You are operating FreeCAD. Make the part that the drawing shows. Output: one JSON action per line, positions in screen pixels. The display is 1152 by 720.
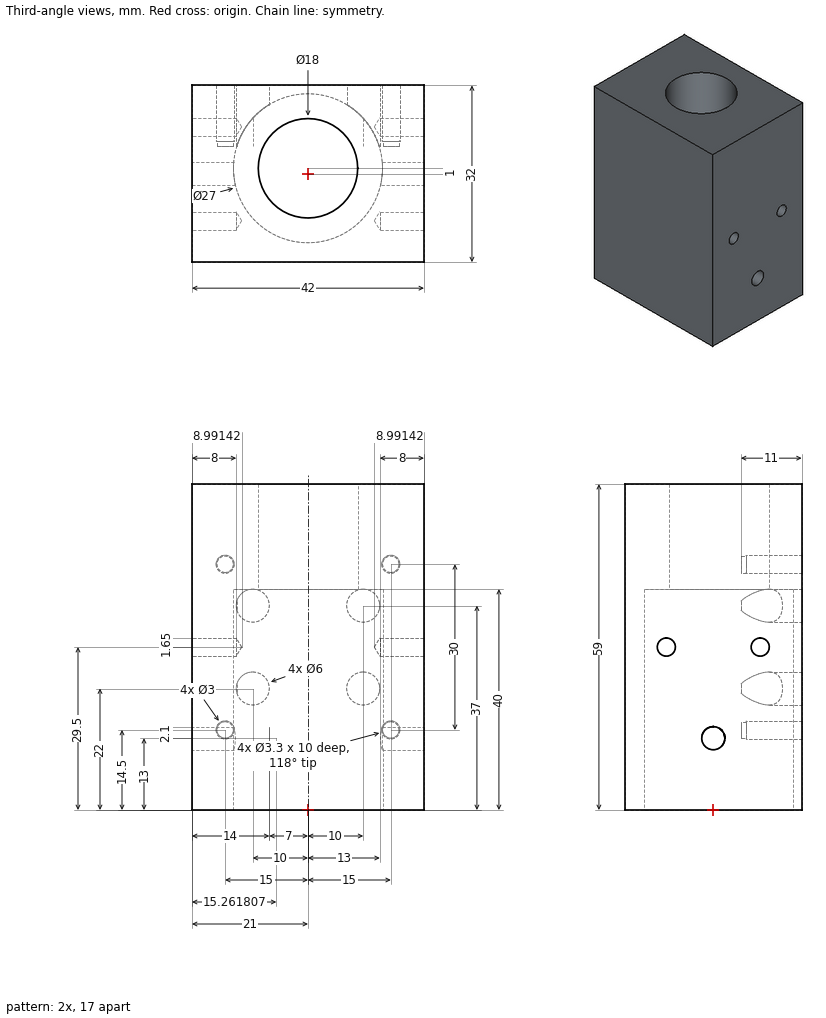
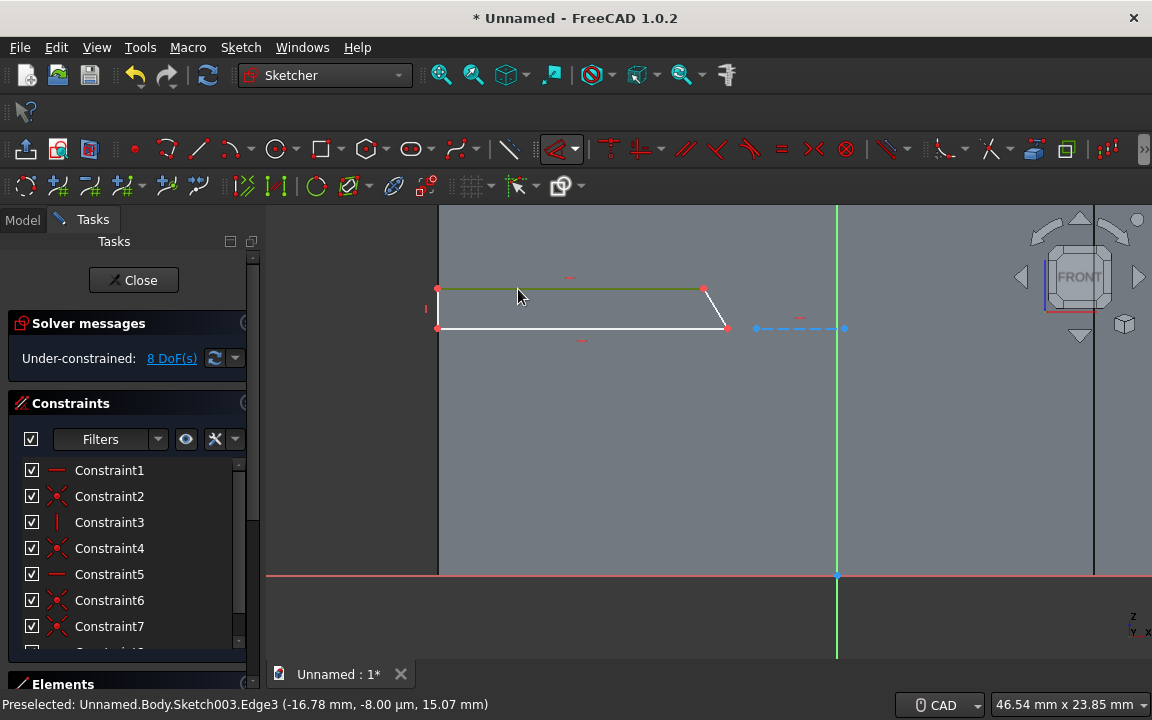
{"action": "key", "text": "l"}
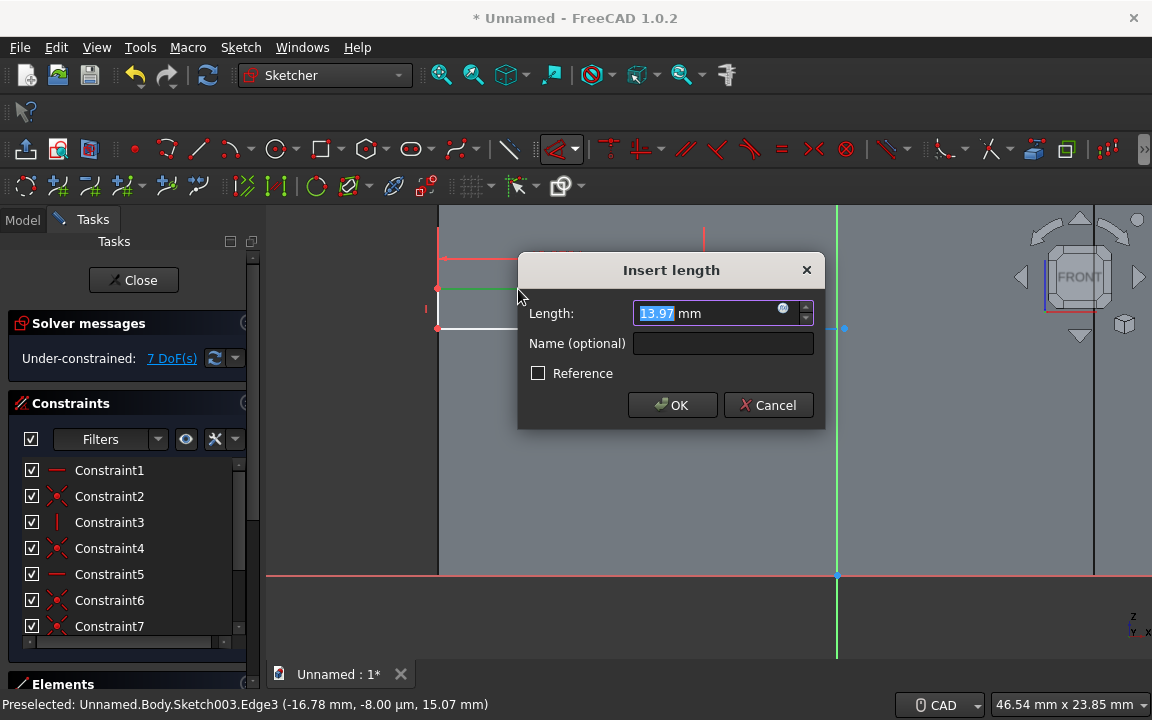
{"action": "type", "text": "14"}
{"action": "key", "text": "Return"}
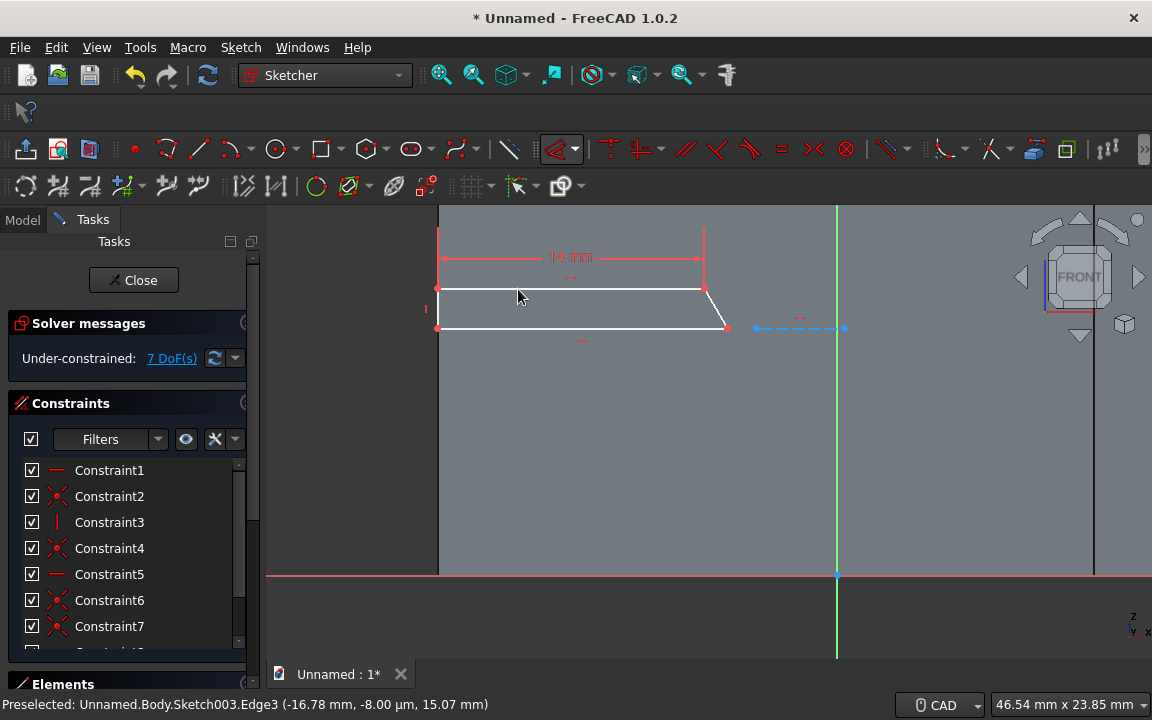
{"action": "left_click", "coordinate": [704, 289]}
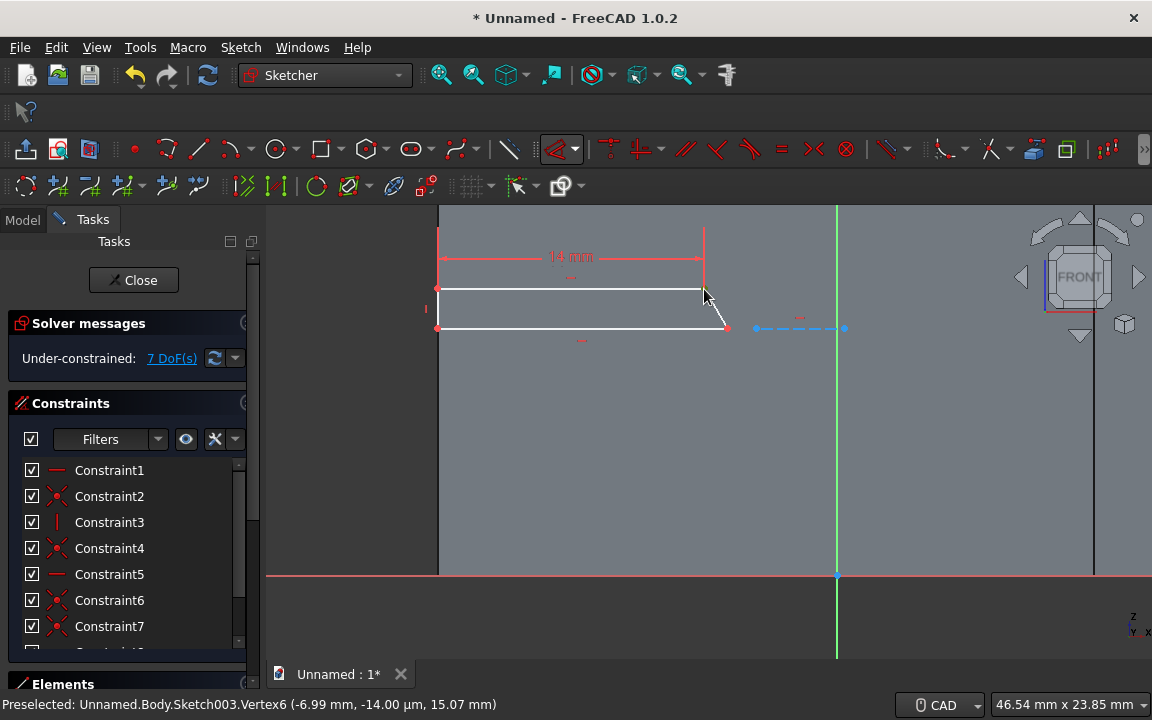
{"action": "key", "text": "l"}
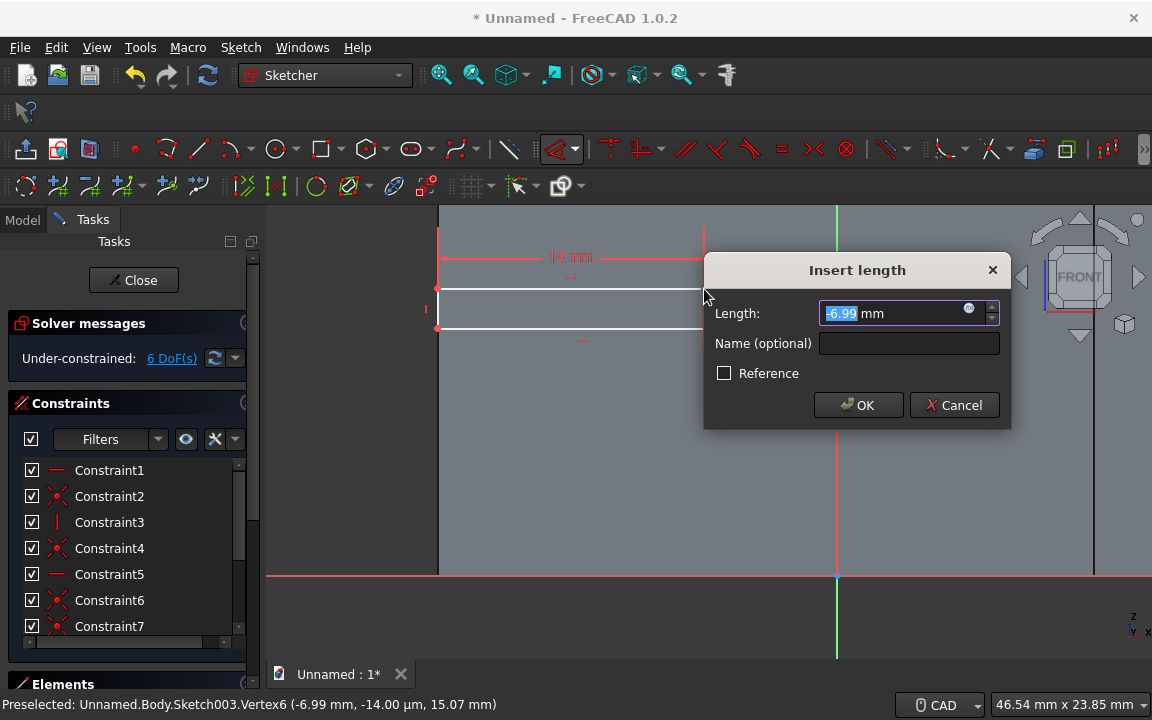
{"action": "type", "text": "-7"}
{"action": "key", "text": "Return"}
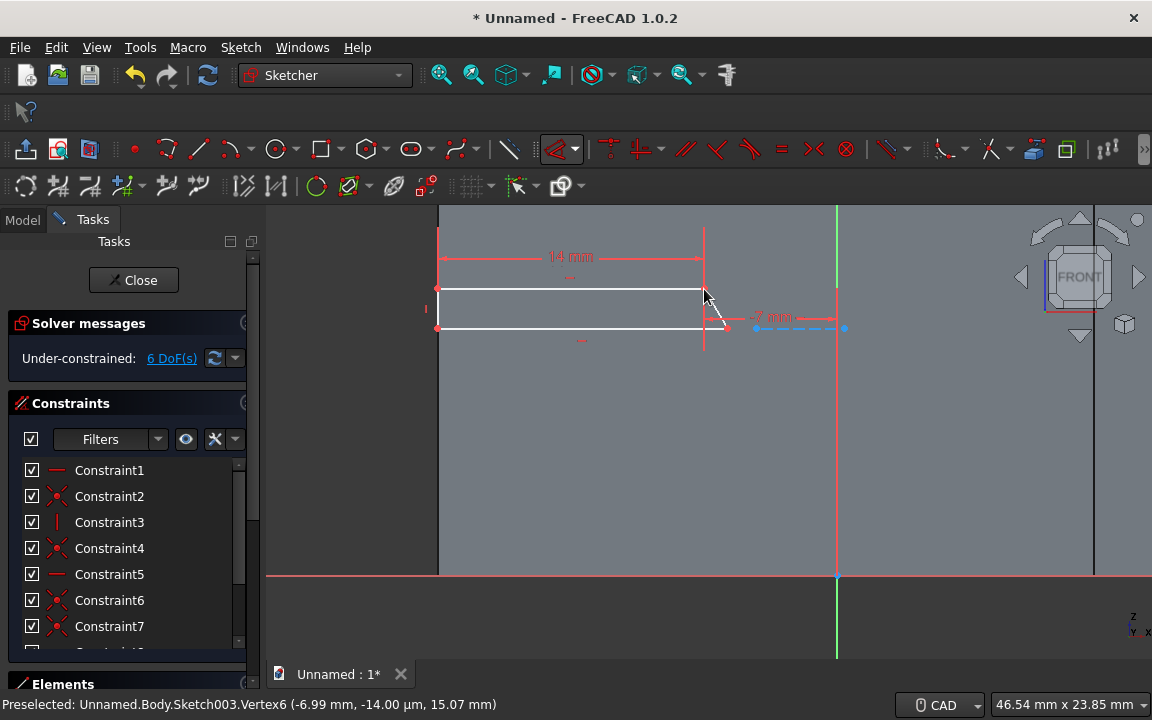
{"action": "left_click", "coordinate": [438, 317]}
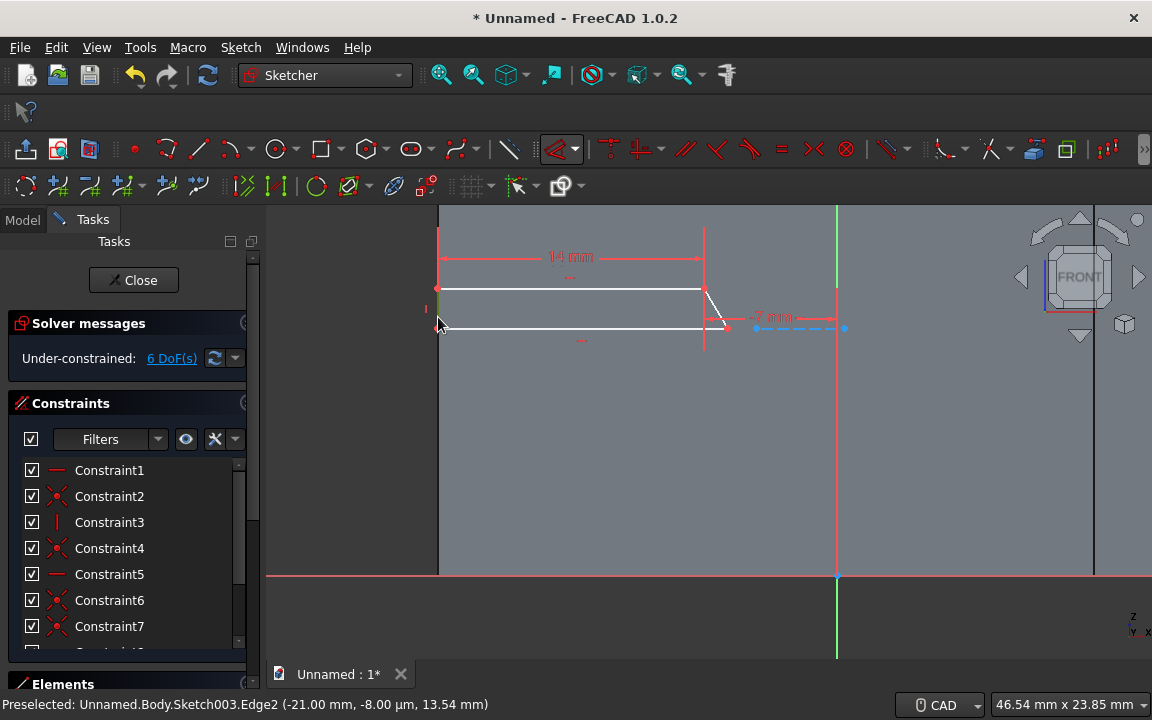
{"action": "key", "text": "i"}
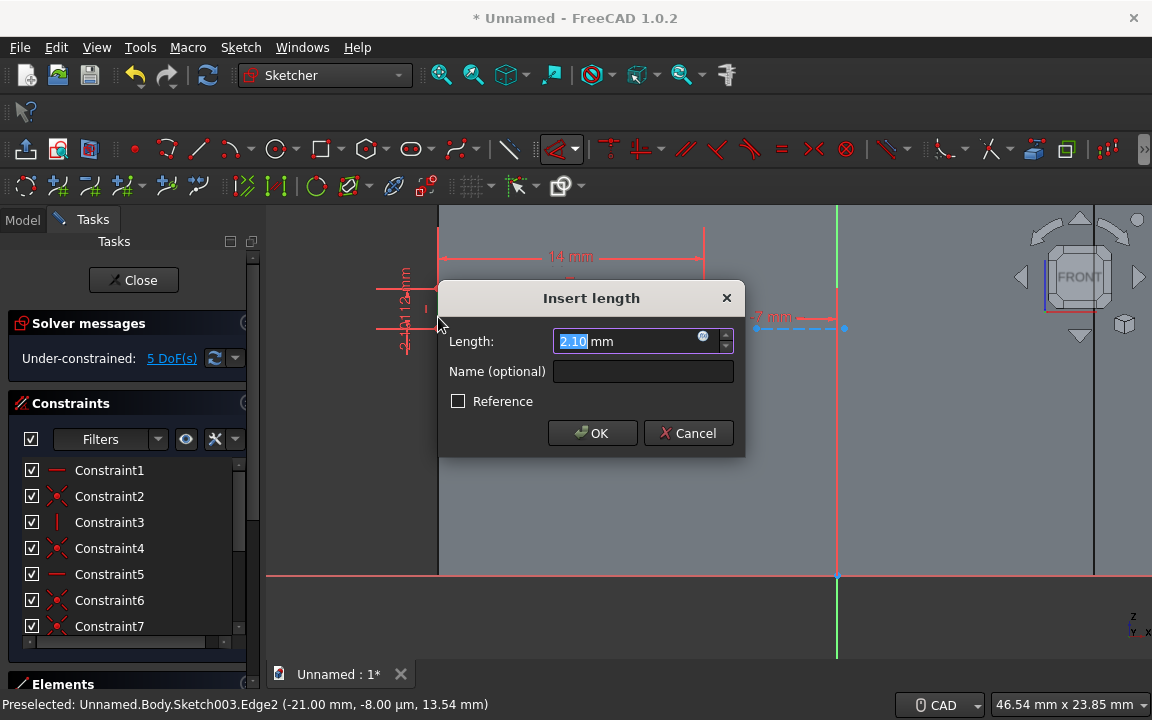
{"action": "type", "text": "2.1"}
{"action": "key", "text": "Return"}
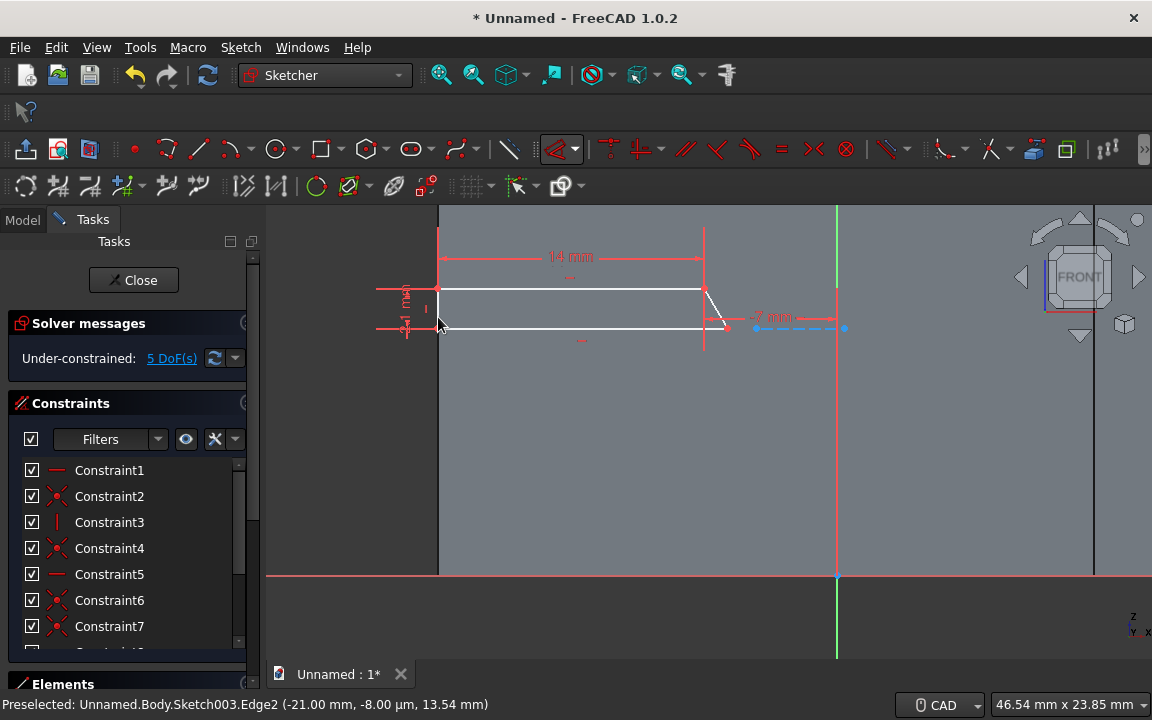
{"action": "left_click", "coordinate": [728, 329]}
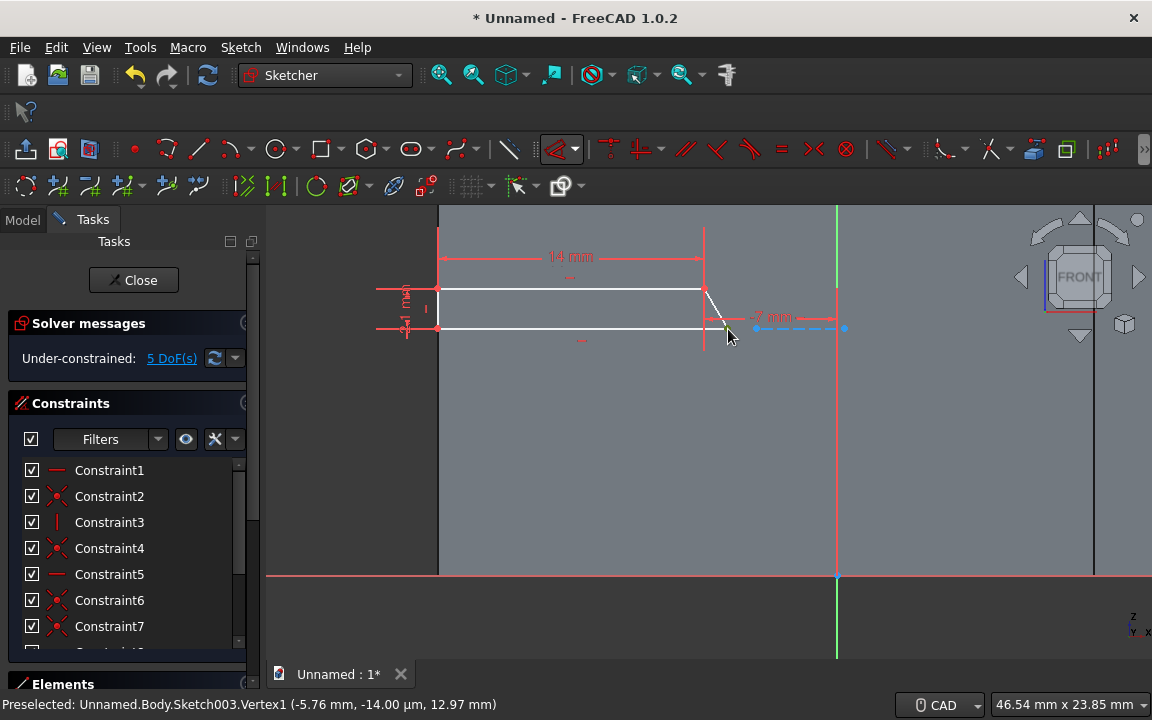
{"action": "key", "text": "i"}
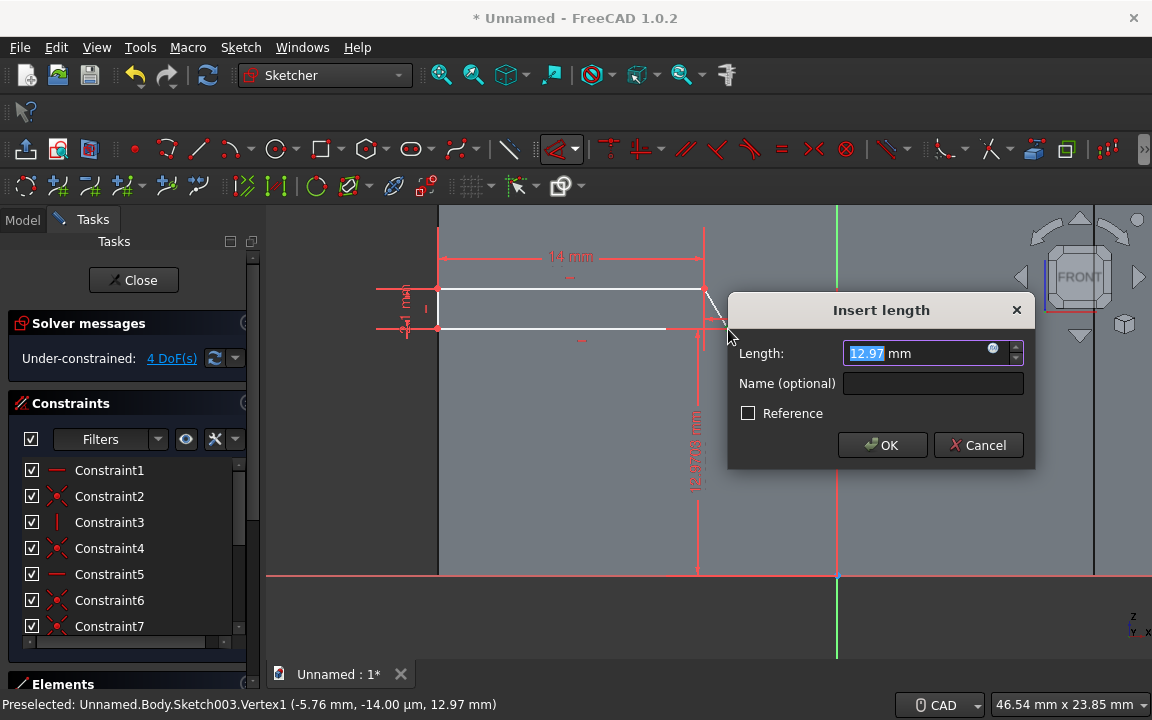
{"action": "type", "text": "13"}
{"action": "key", "text": "Return"}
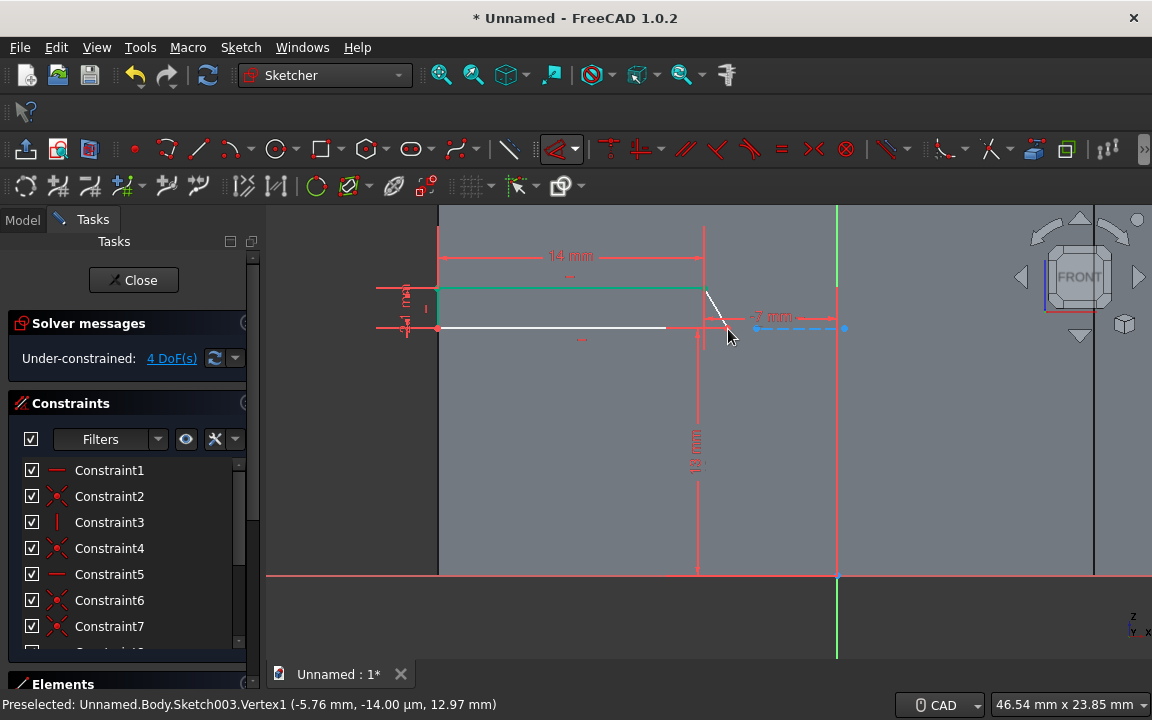
{"action": "left_click", "coordinate": [757, 329]}